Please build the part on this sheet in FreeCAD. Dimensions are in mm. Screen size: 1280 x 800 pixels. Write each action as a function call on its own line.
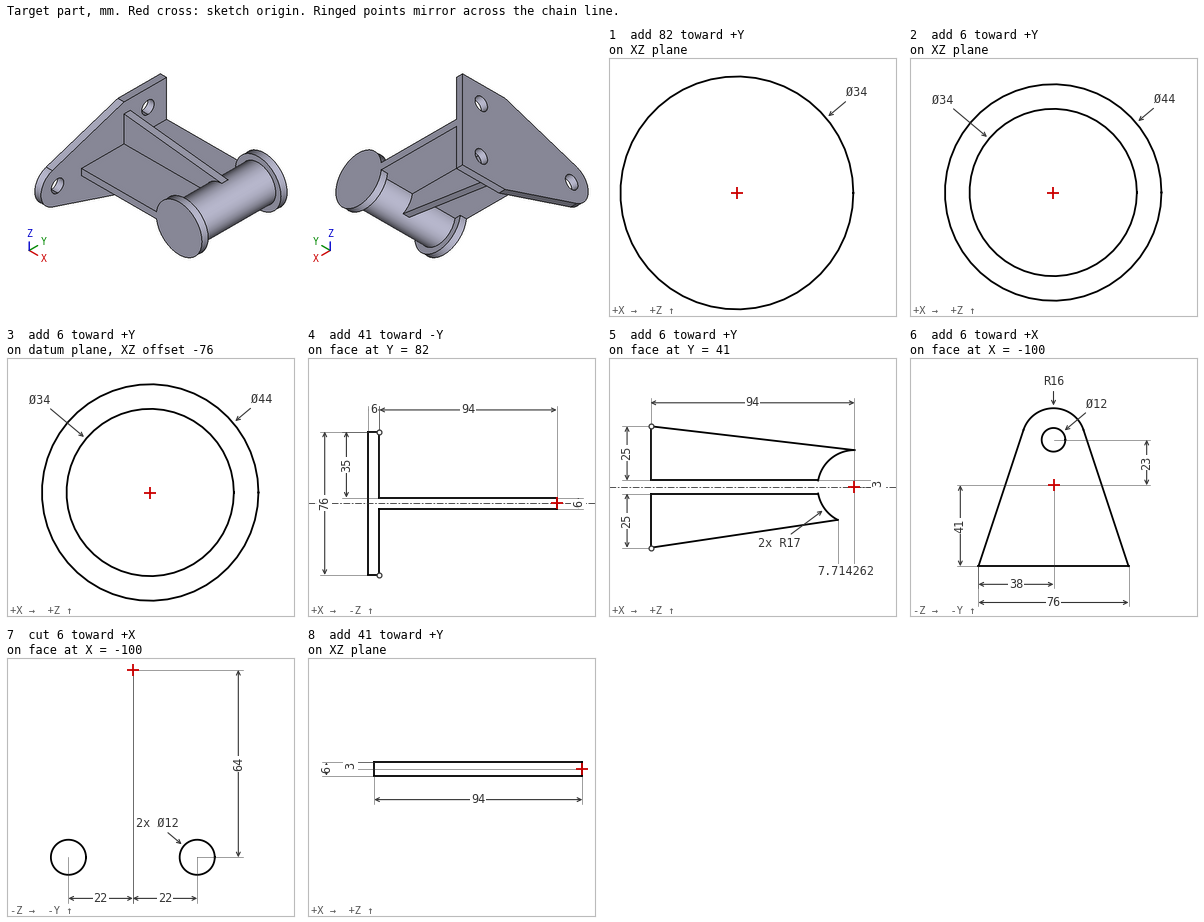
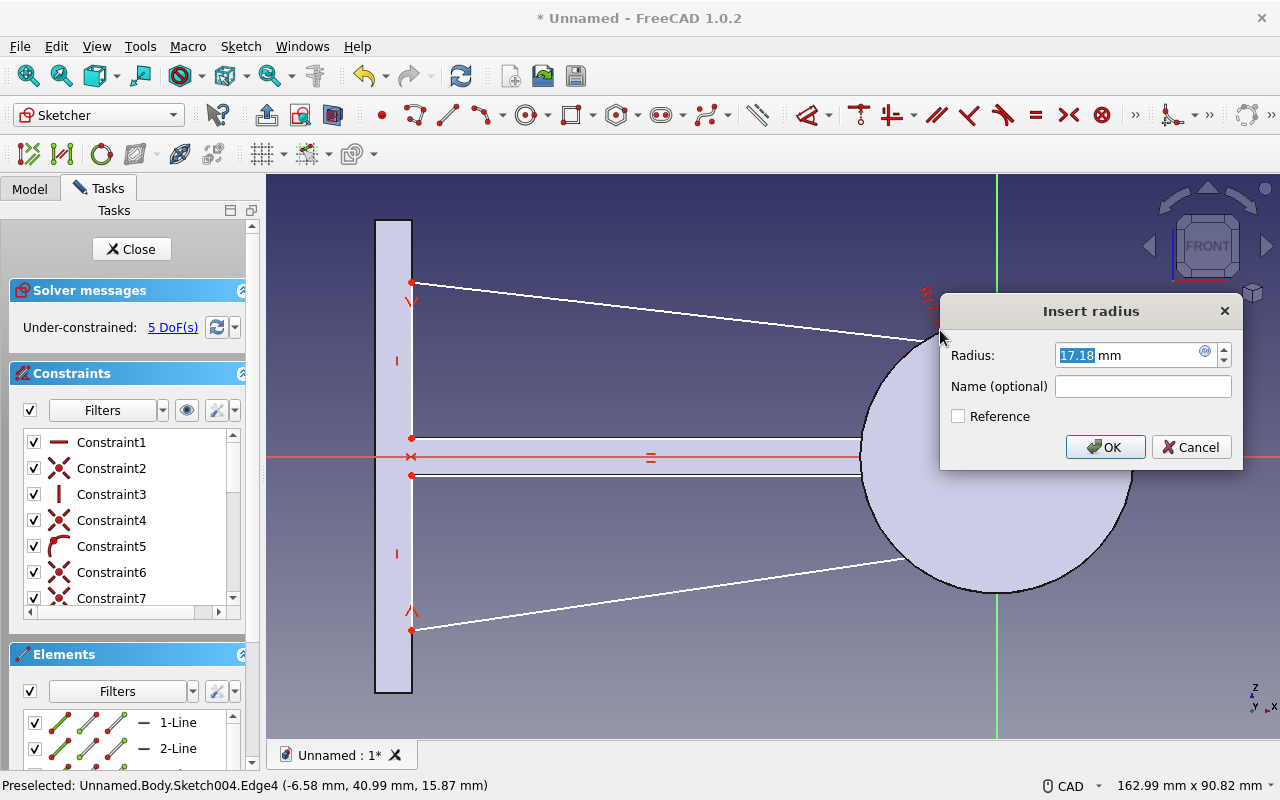
text(17)
key(Return)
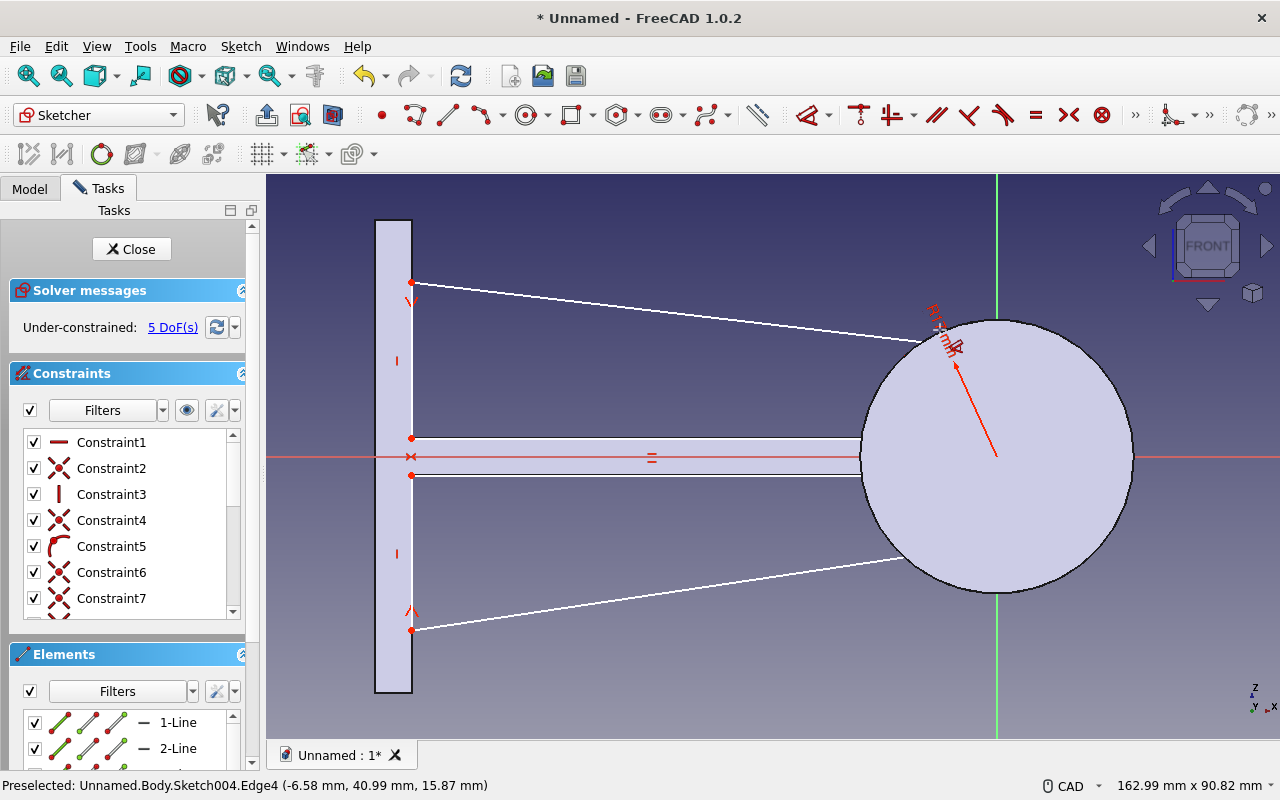
click(412, 392)
click(378, 361)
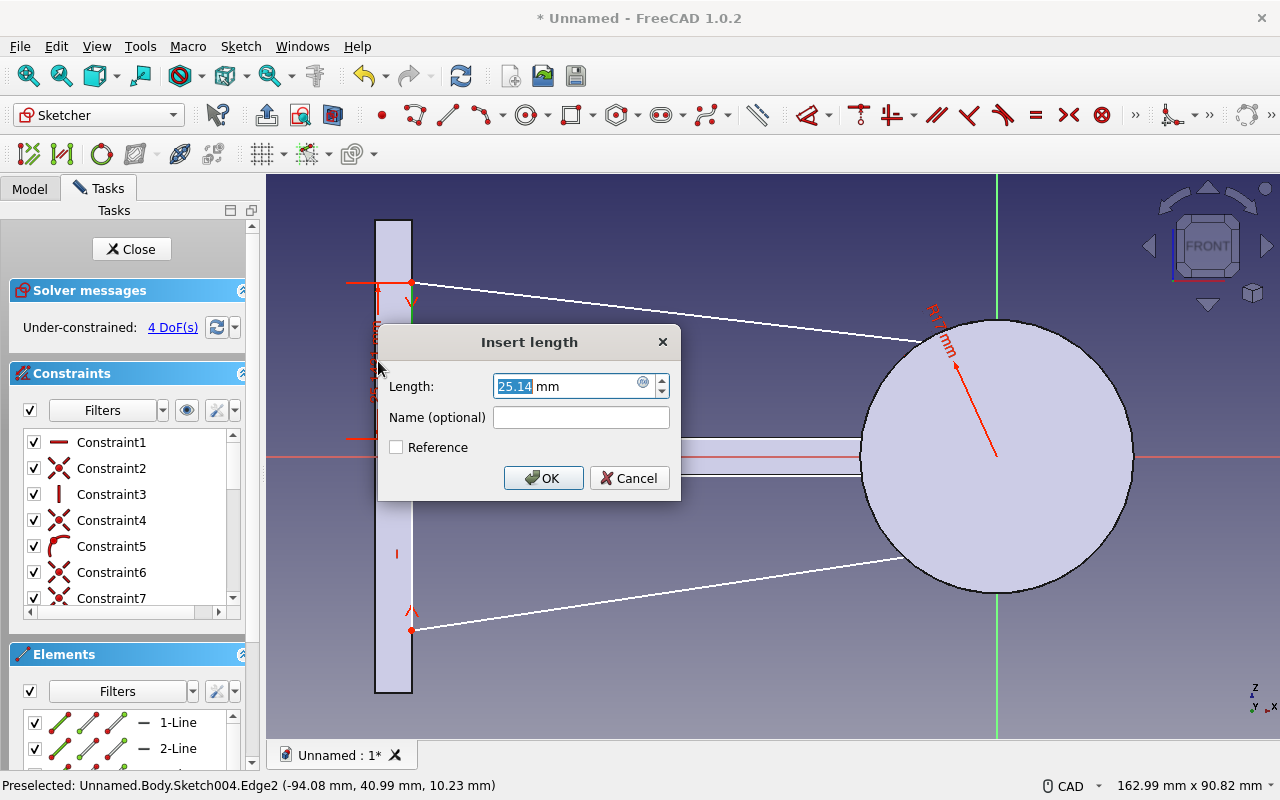
text(25)
key(Return)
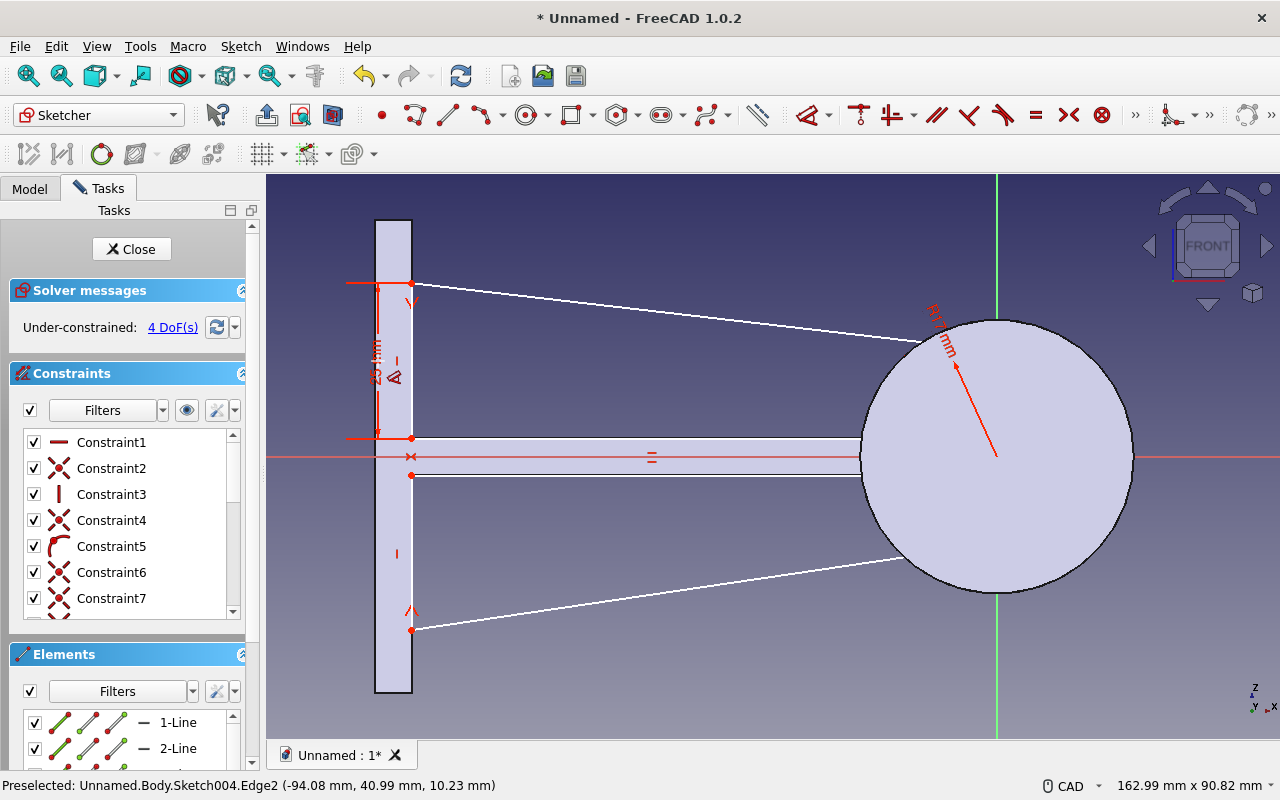
click(412, 584)
click(378, 553)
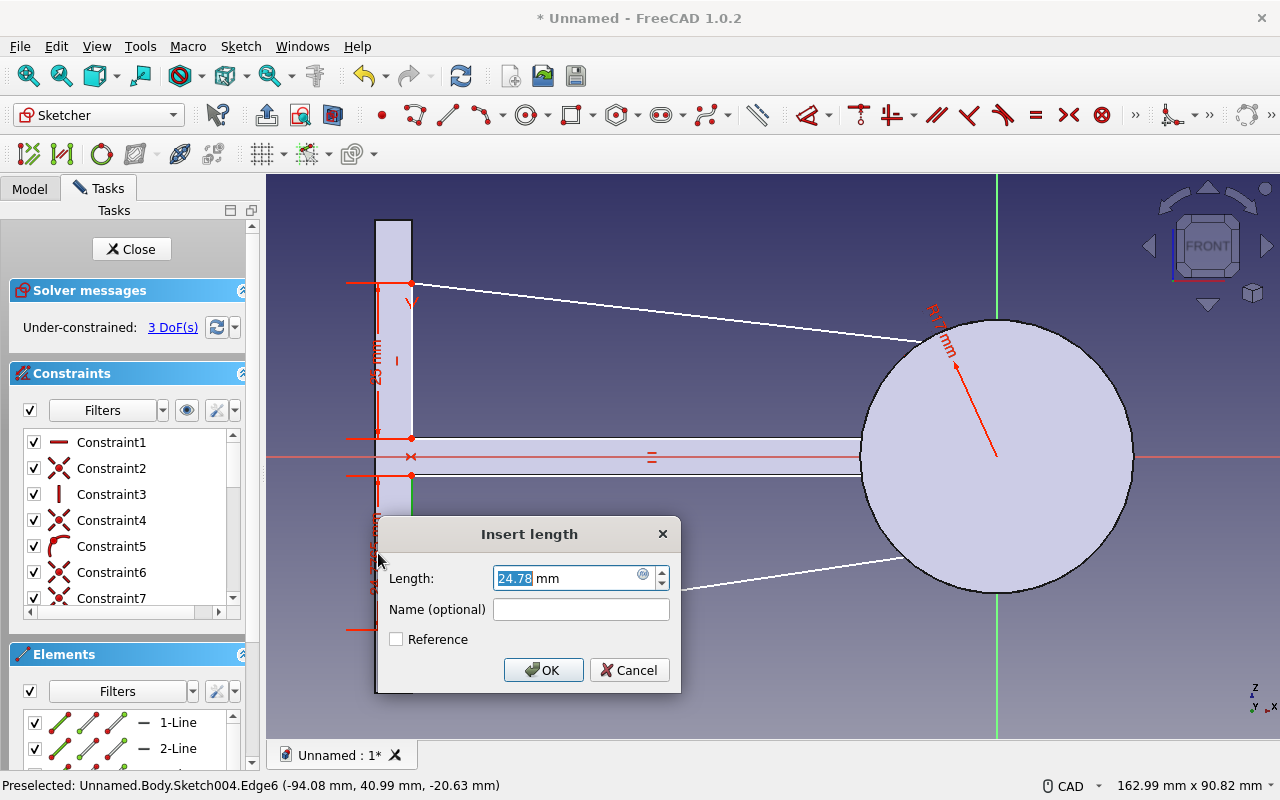
text(25)
key(Return)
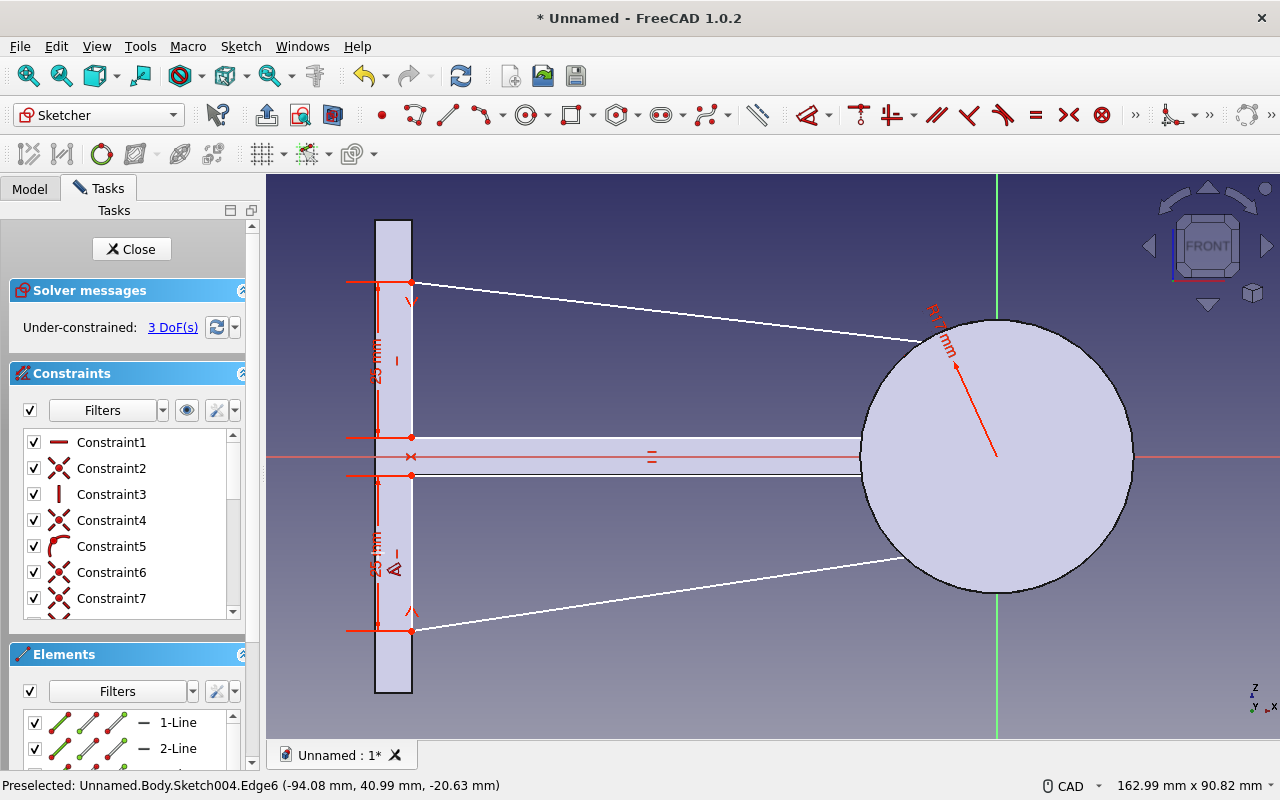
scroll(893, 438, up, 4)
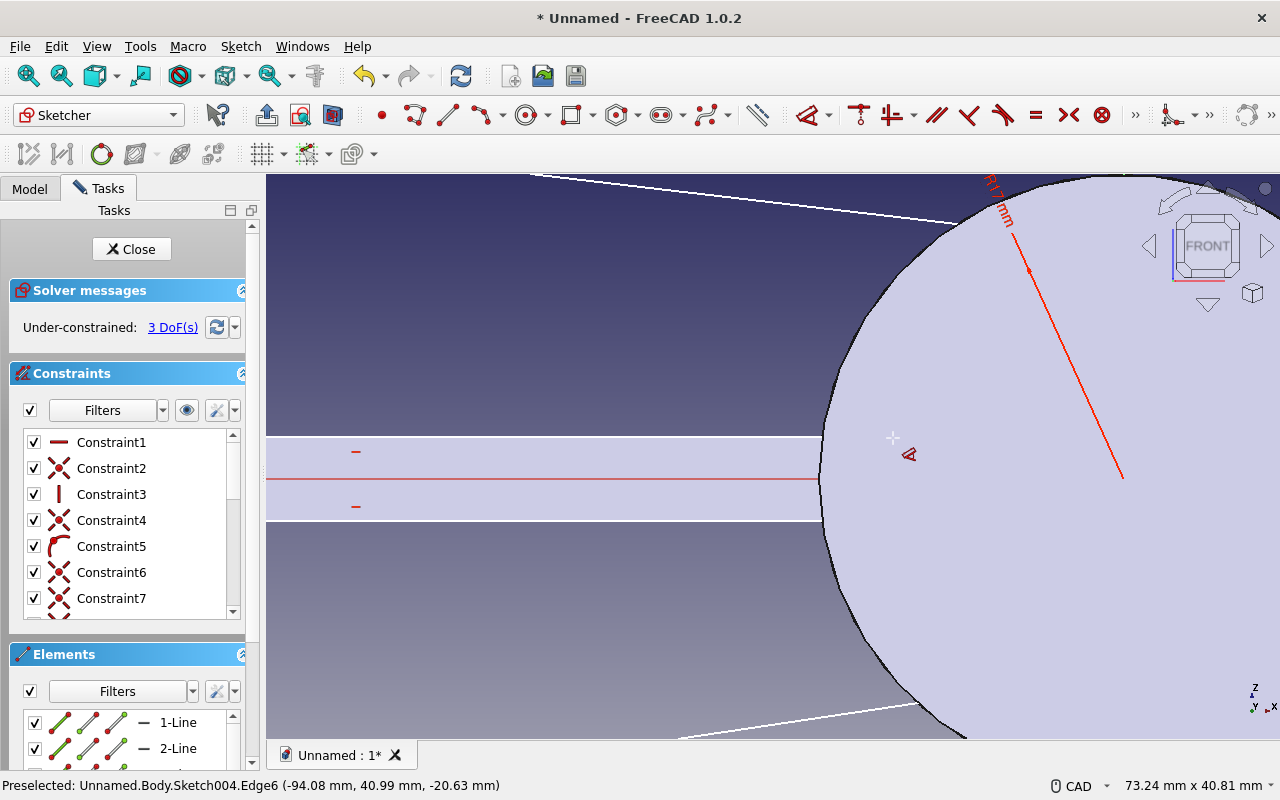
click(892, 437)
click(858, 458)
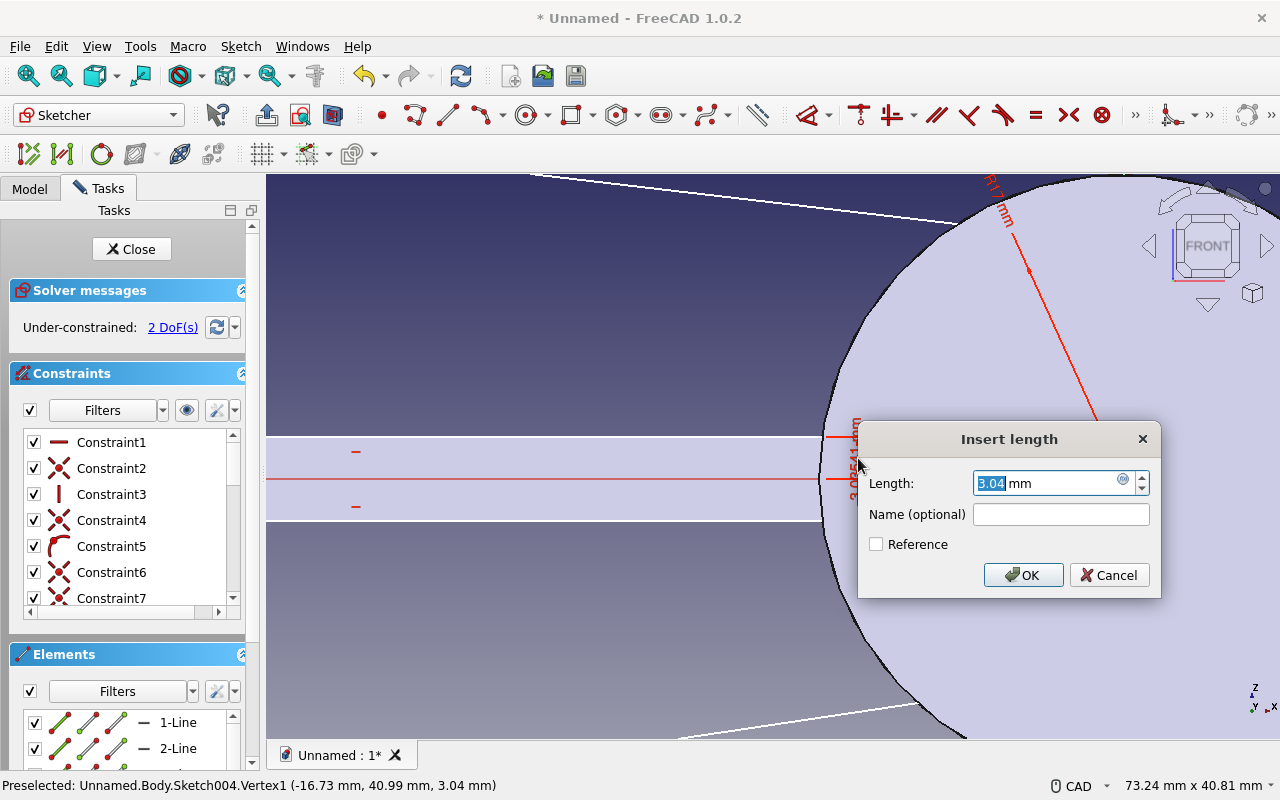
text(3)
key(Return)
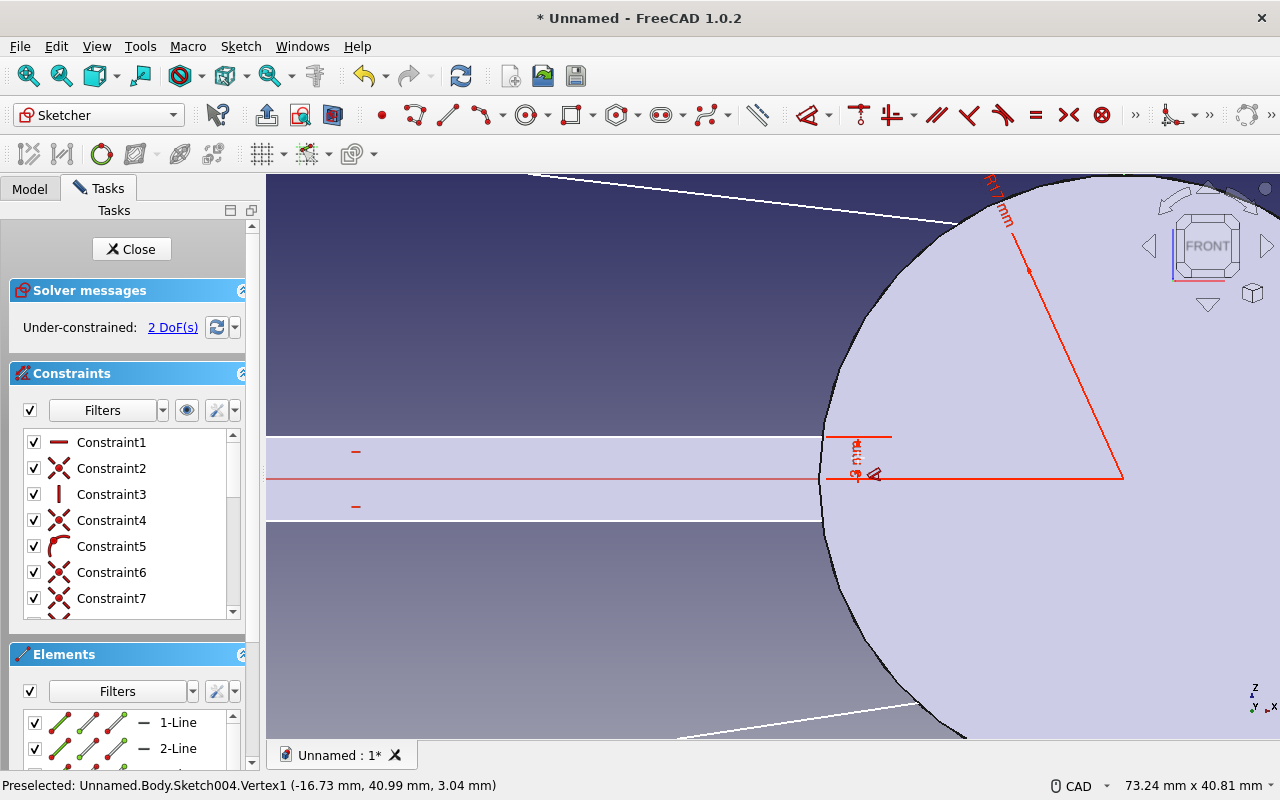
scroll(894, 438, down, 4)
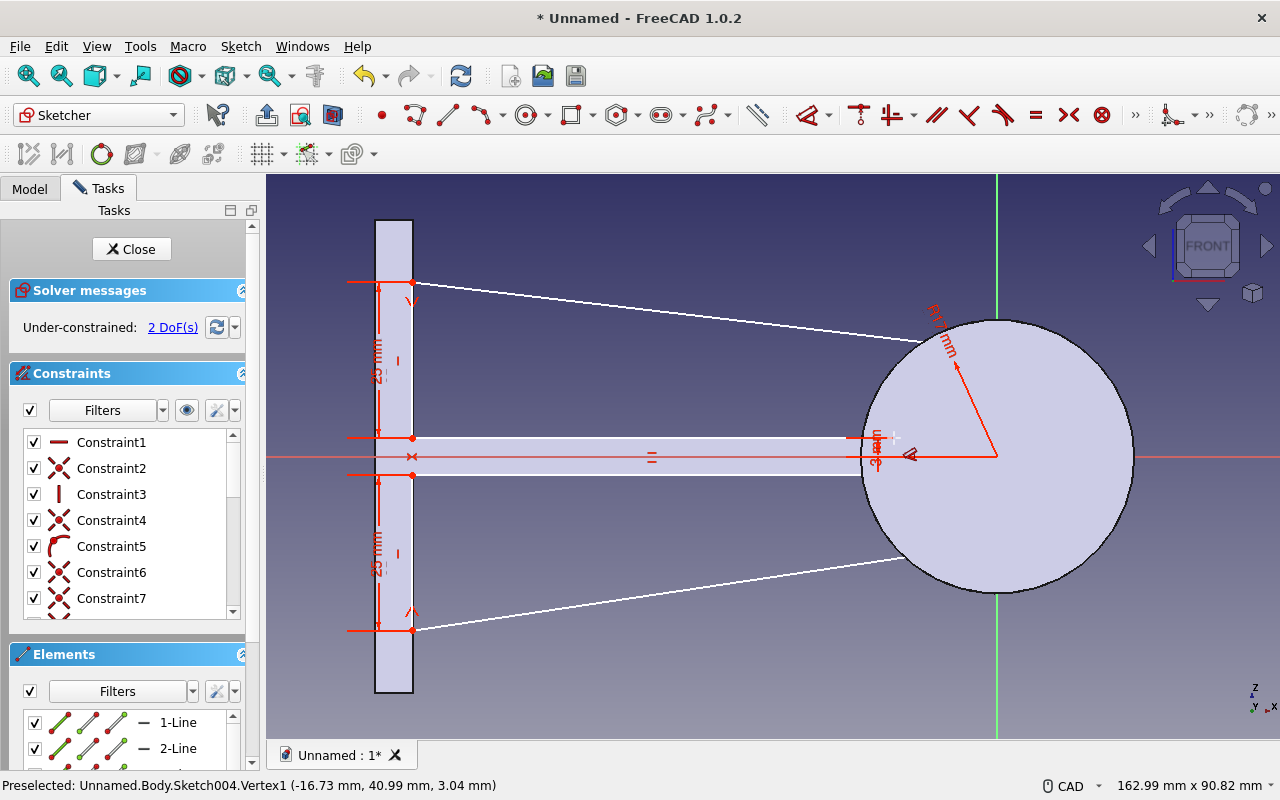
click(412, 438)
click(705, 404)